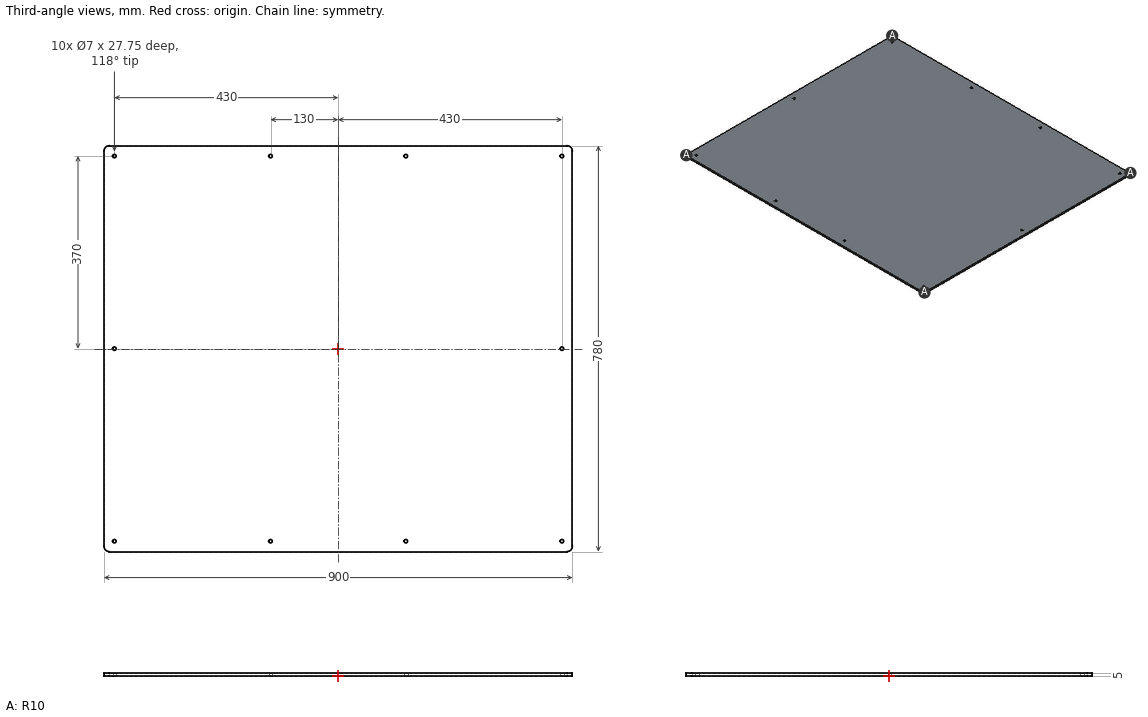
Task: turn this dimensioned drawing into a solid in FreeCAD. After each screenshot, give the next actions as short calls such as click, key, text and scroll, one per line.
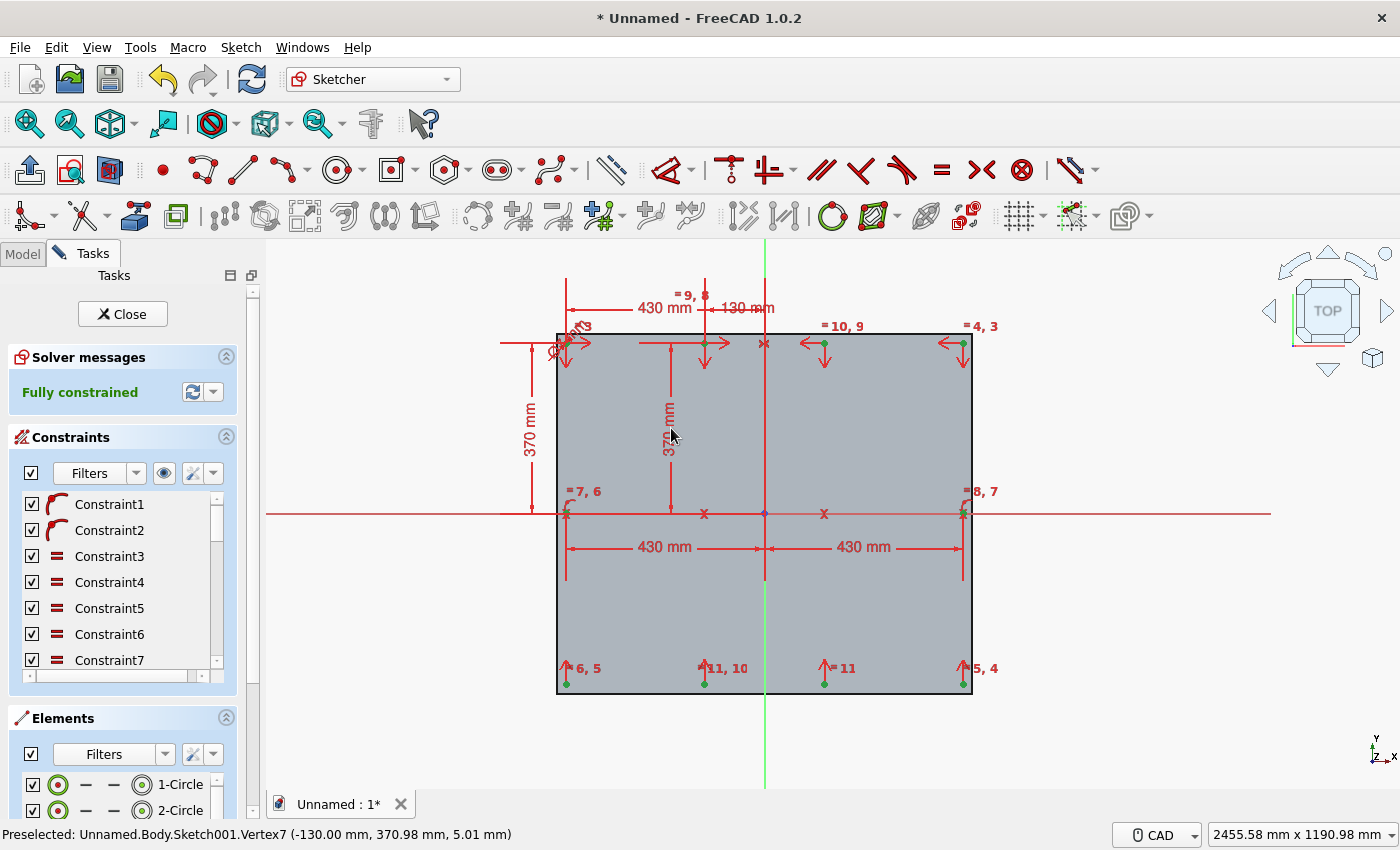
click(123, 314)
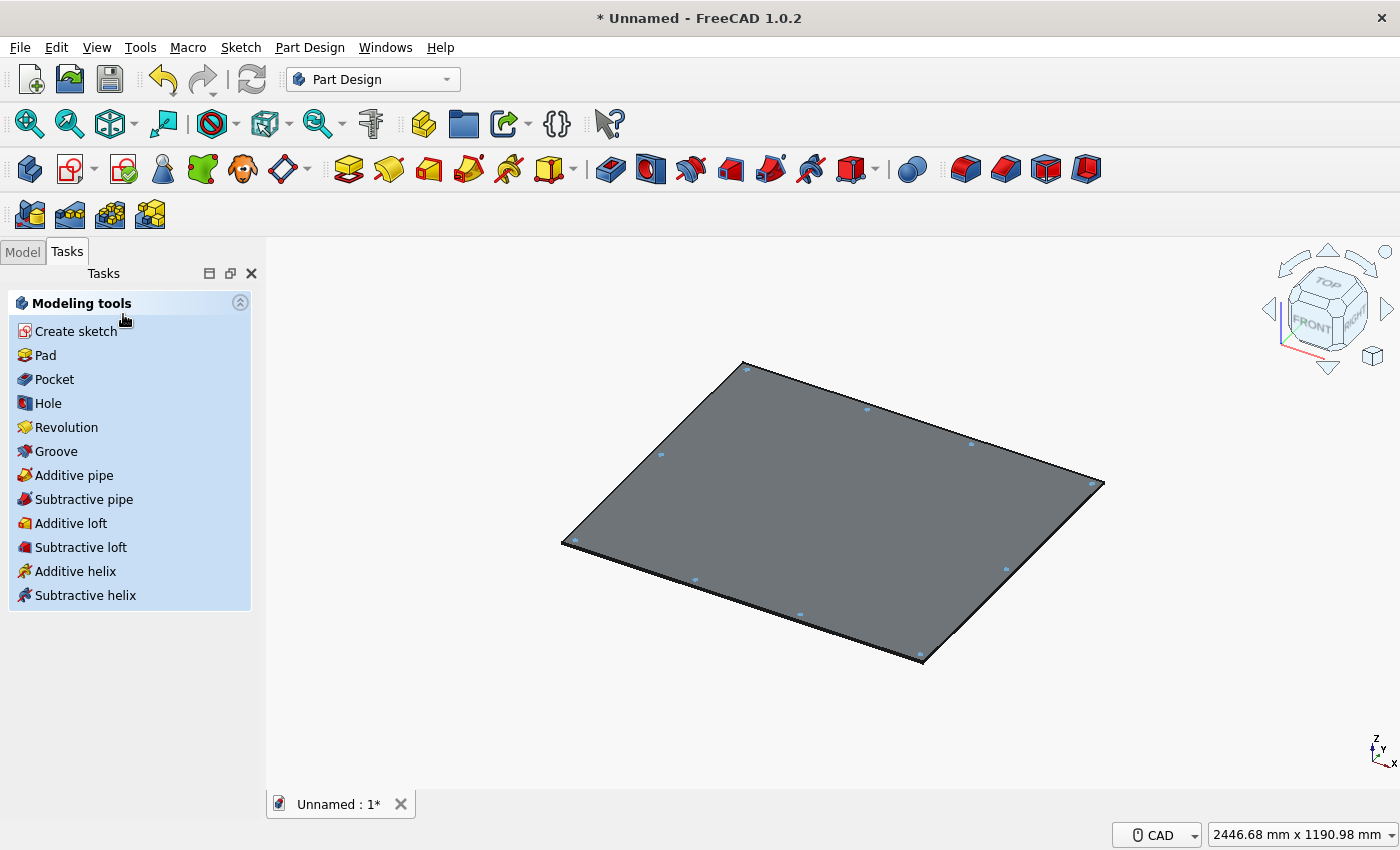
click(652, 170)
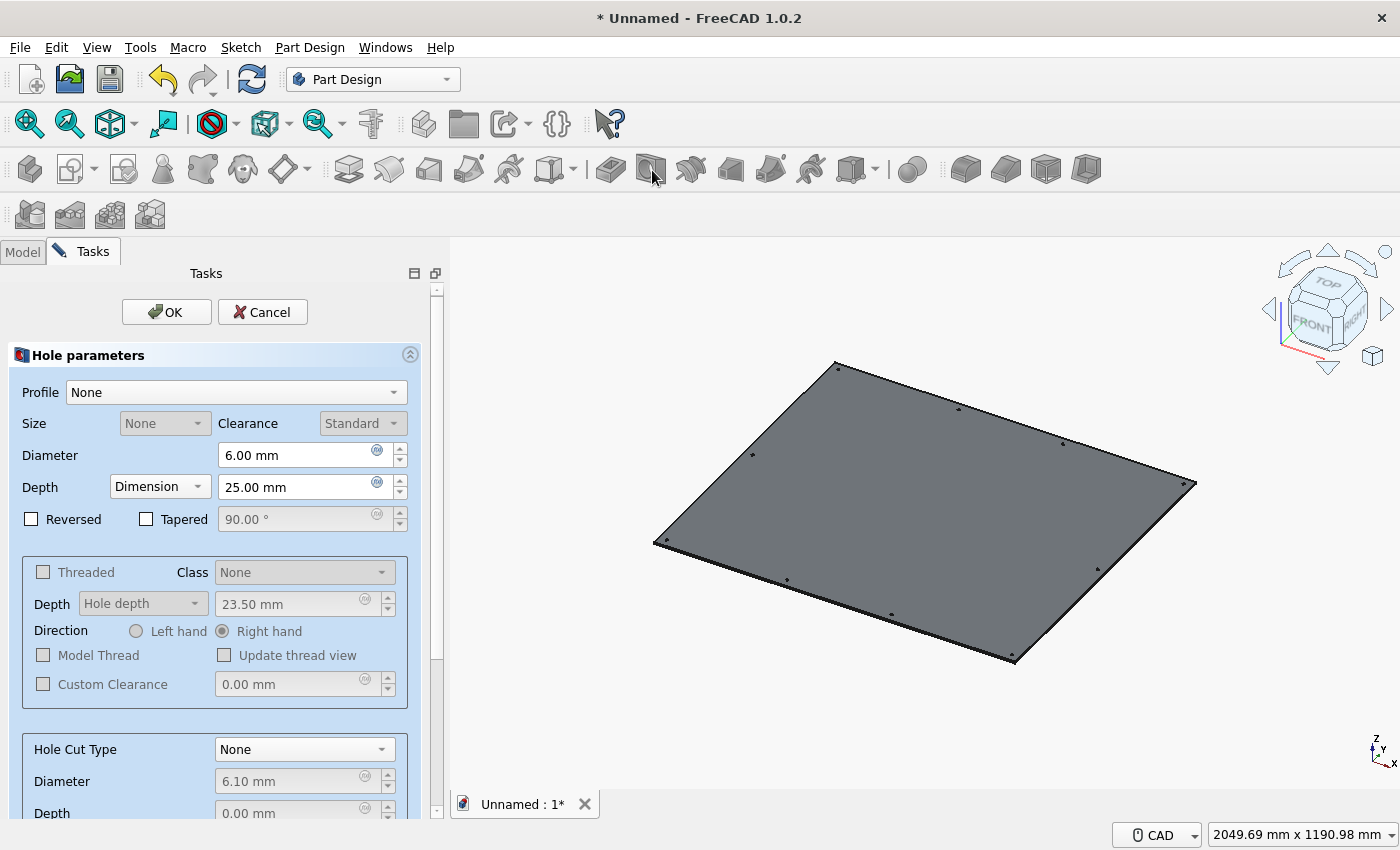
triple_click(305, 455)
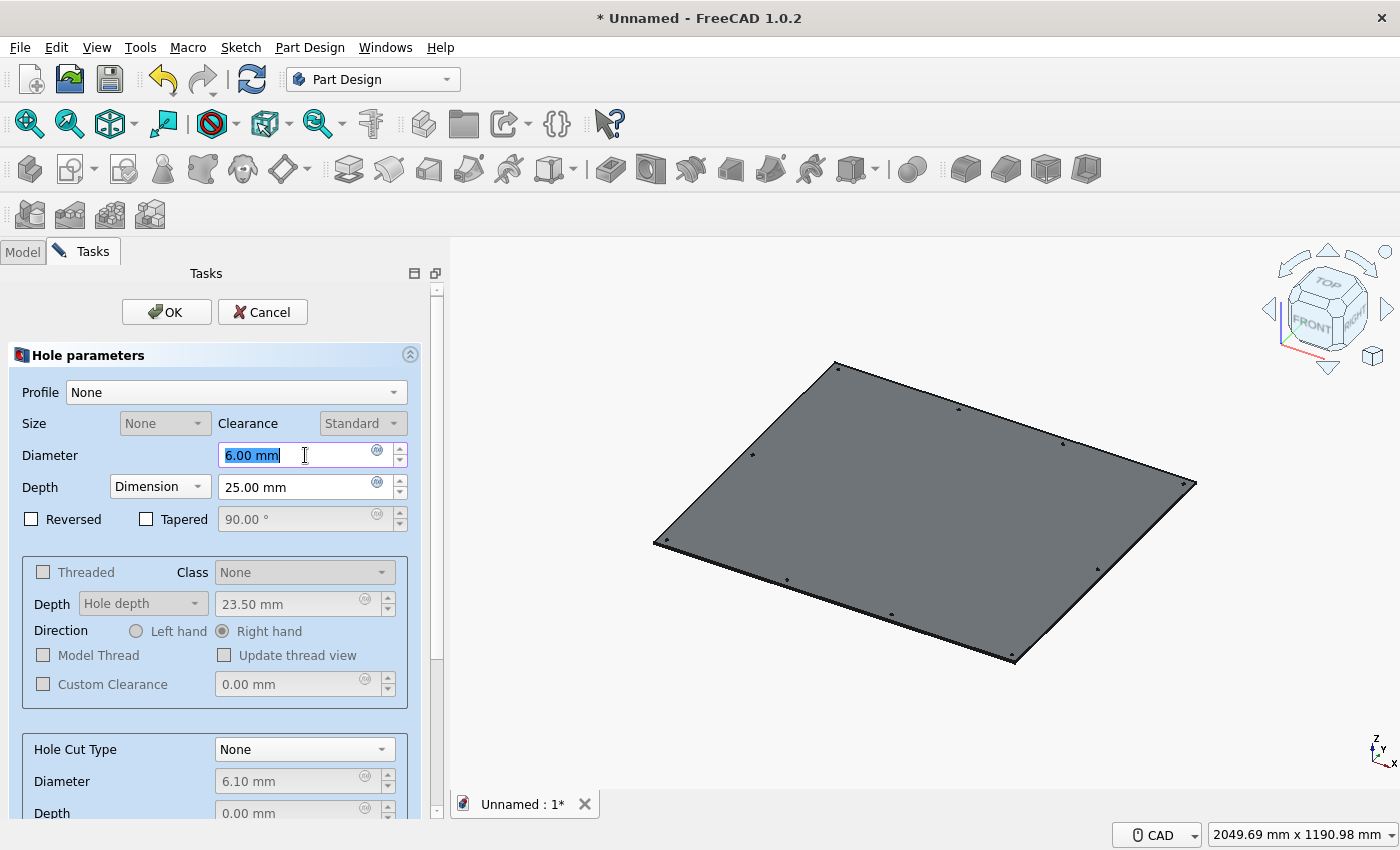
text(7)
key(Tab)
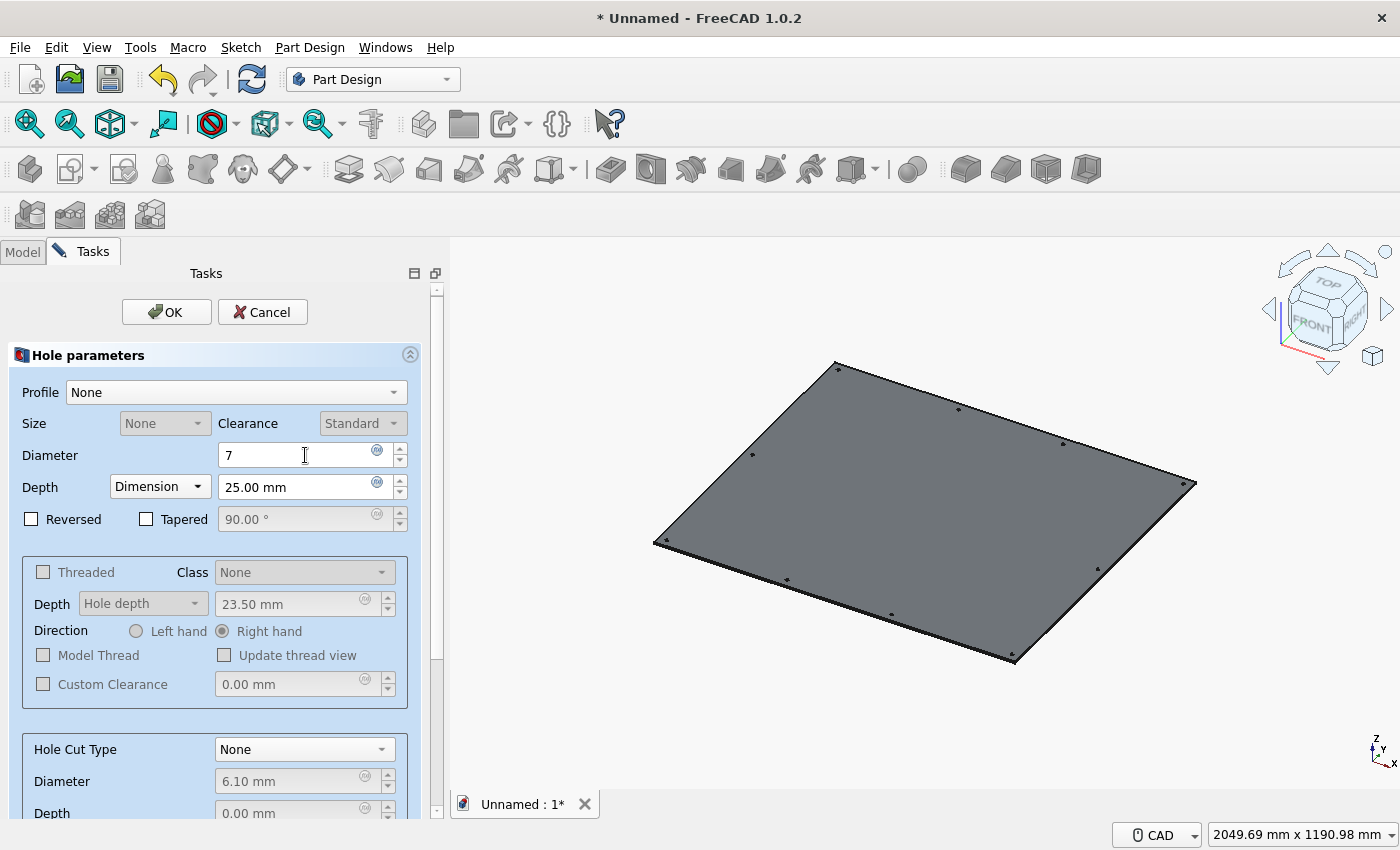
triple_click(305, 487)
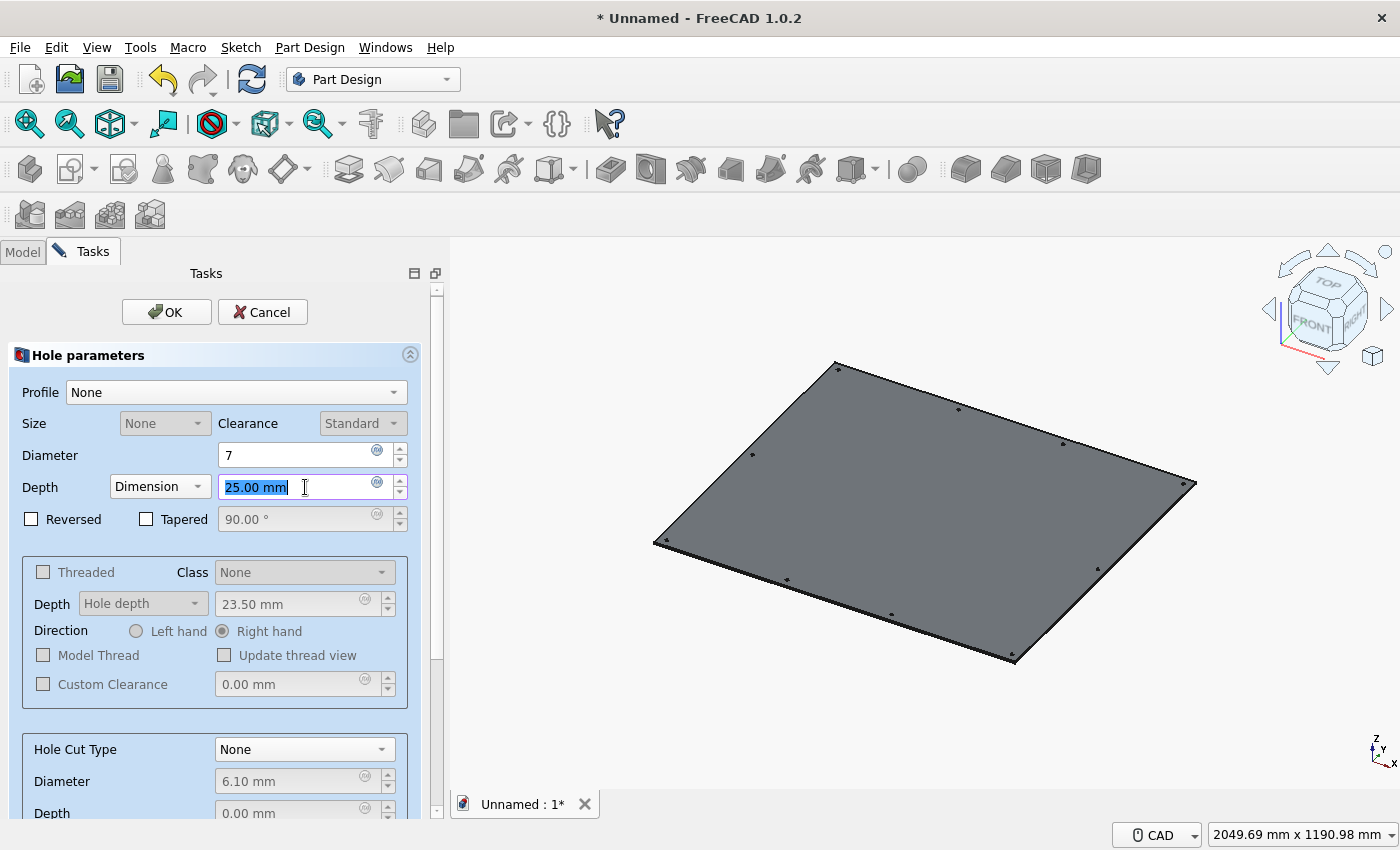
text(27.75)
key(Tab)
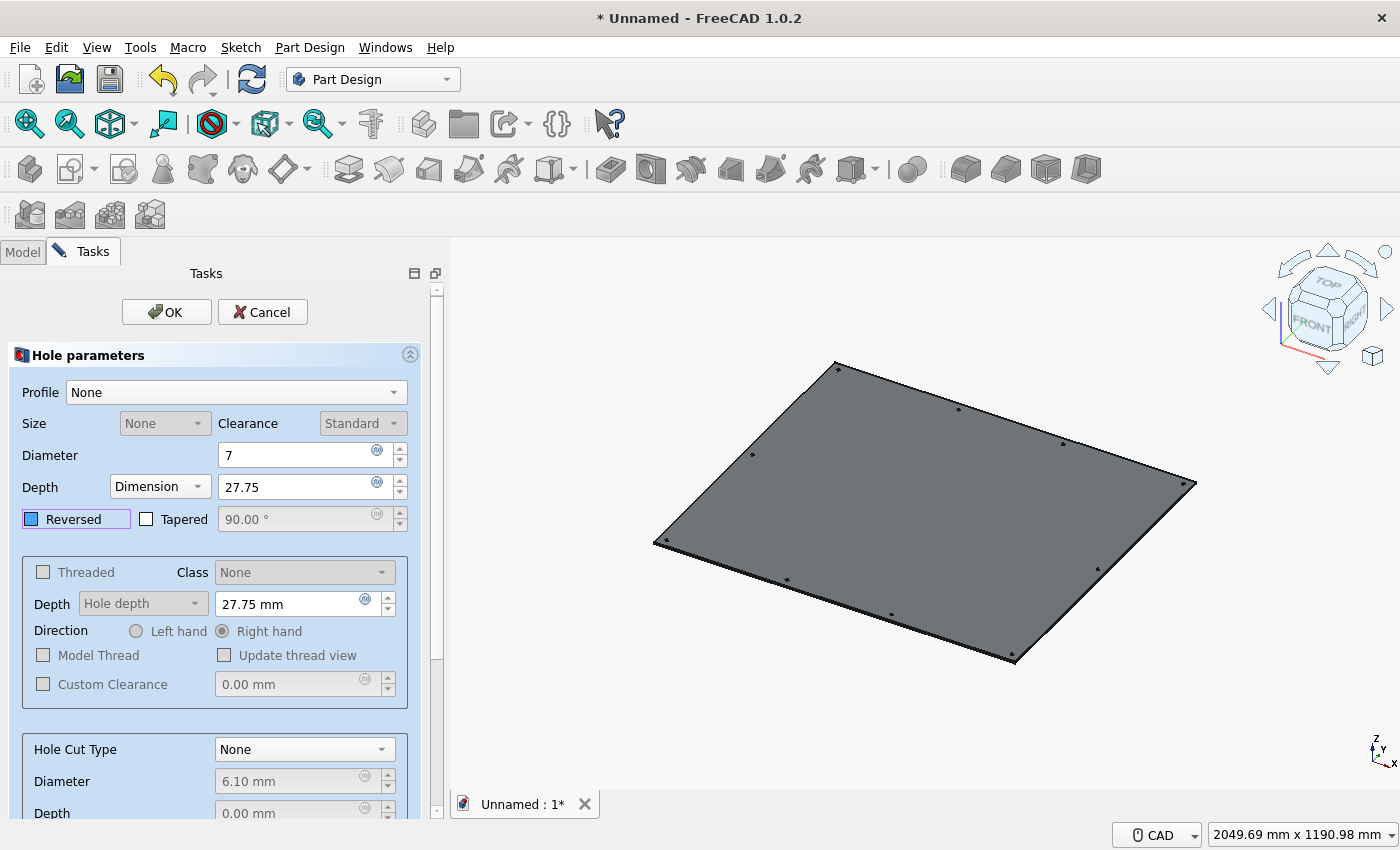
click(167, 312)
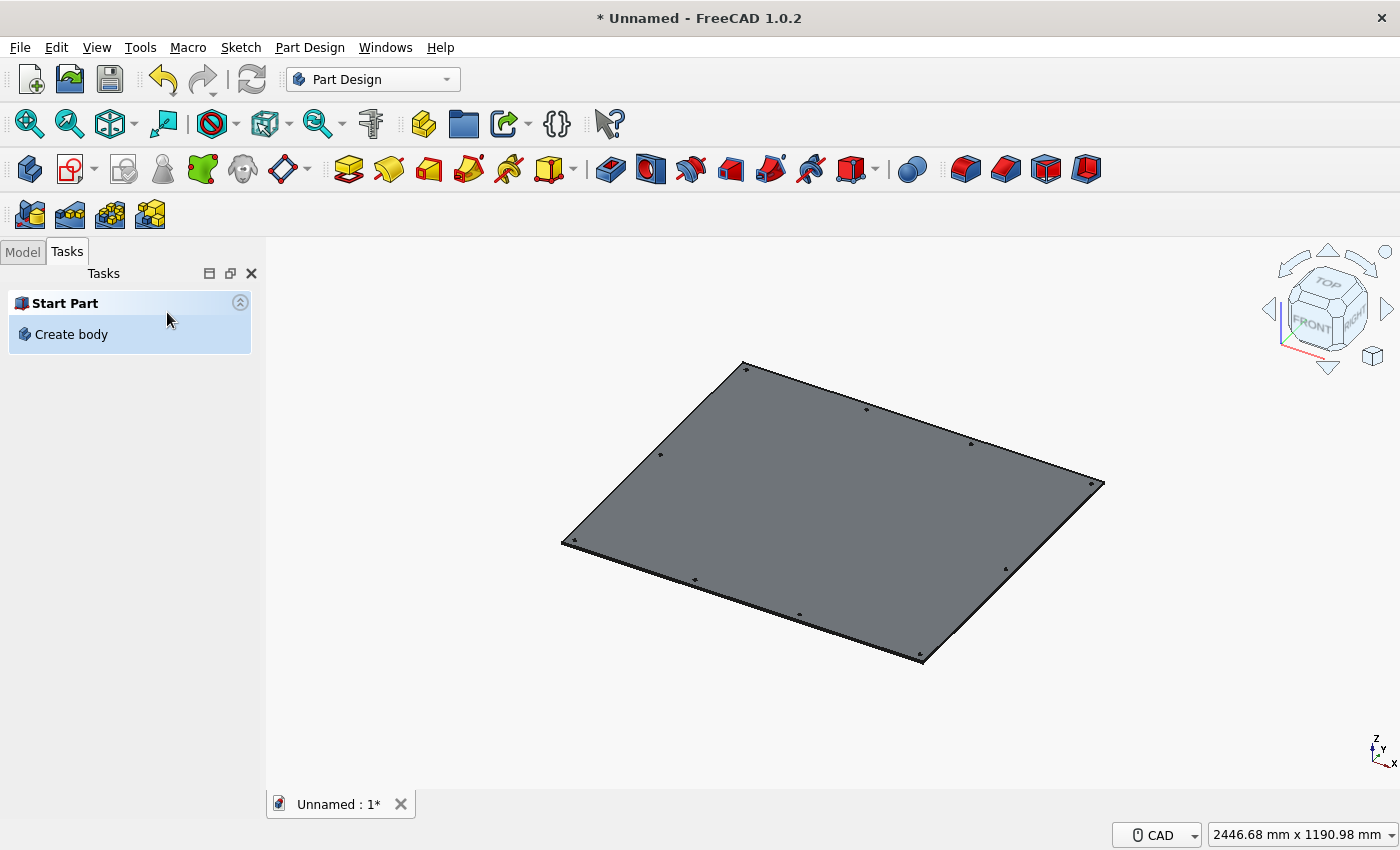
scroll(923, 662, up, 15)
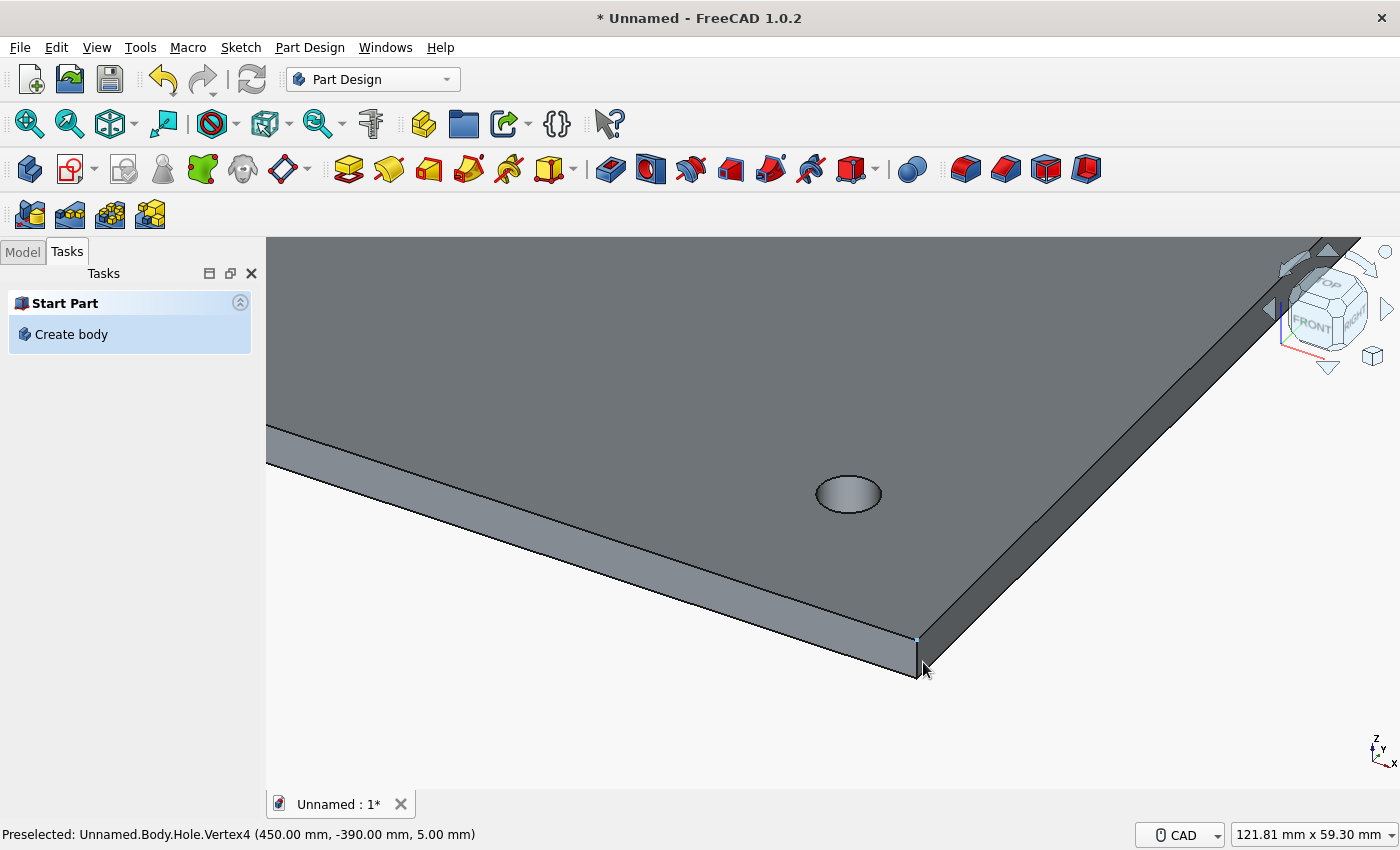
click(917, 658)